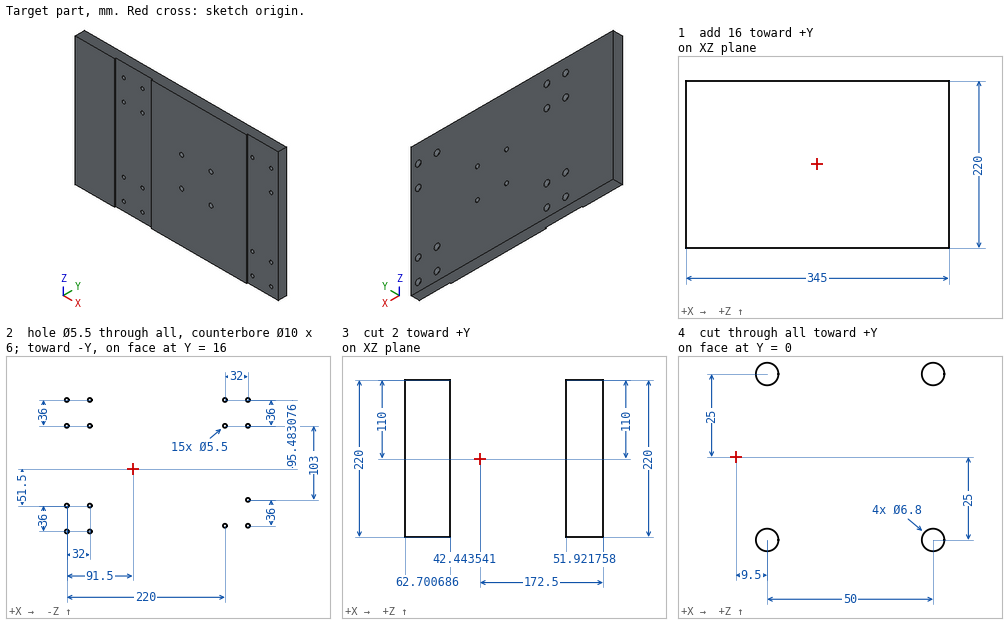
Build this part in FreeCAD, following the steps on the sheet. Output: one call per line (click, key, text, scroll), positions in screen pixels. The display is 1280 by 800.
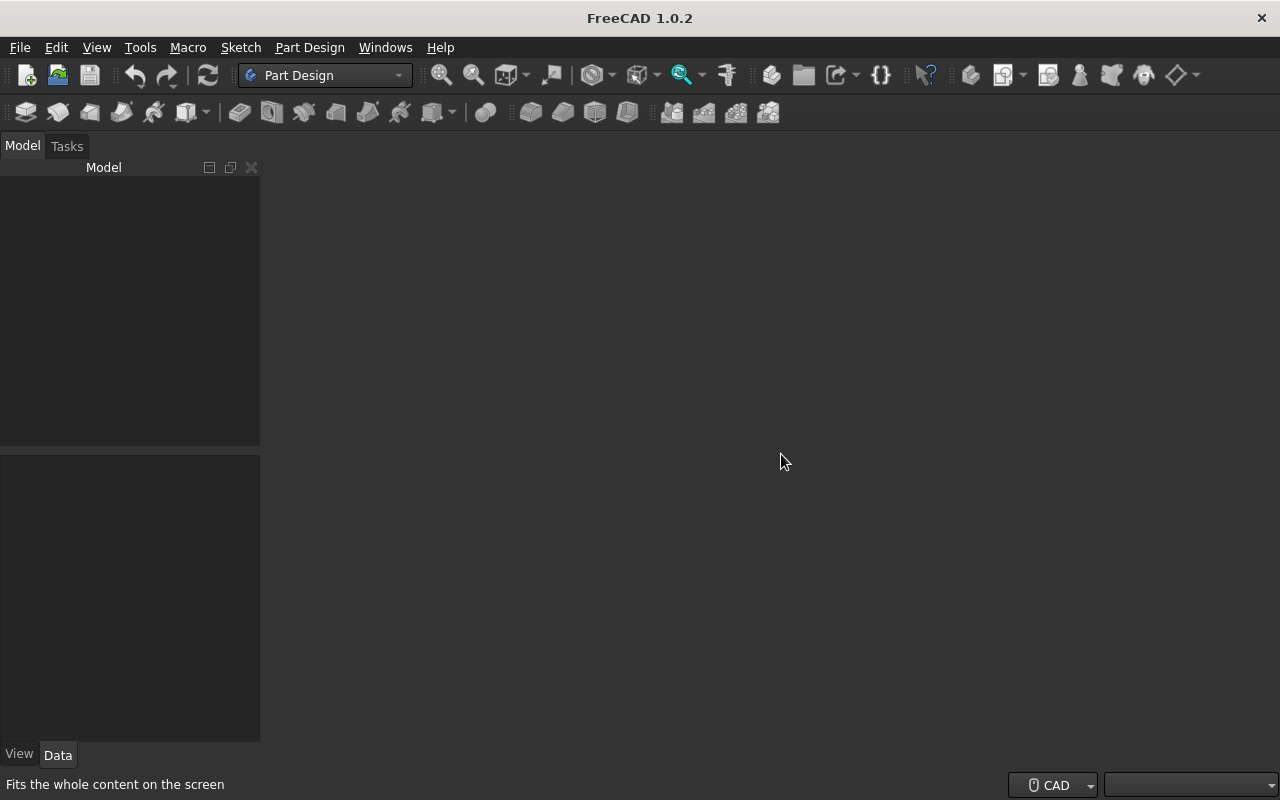
key(ctrl+n)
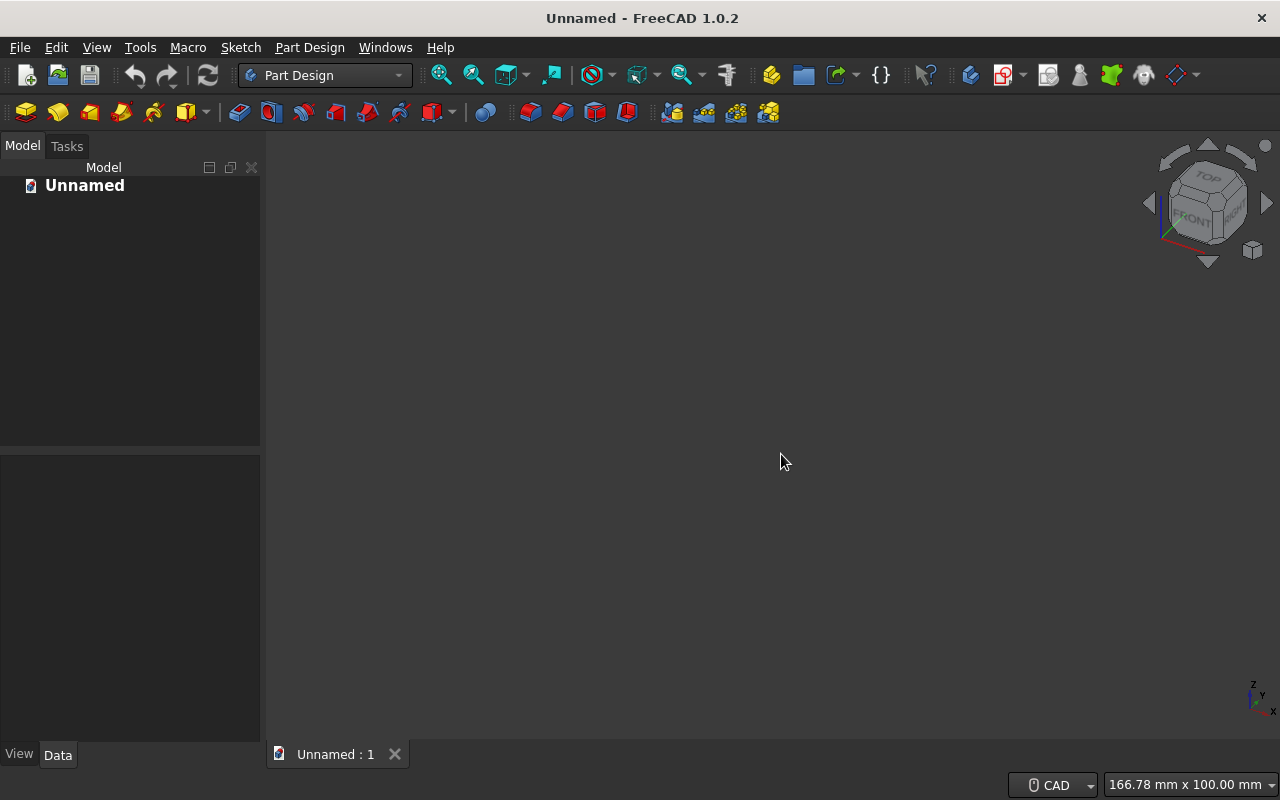
click(1004, 76)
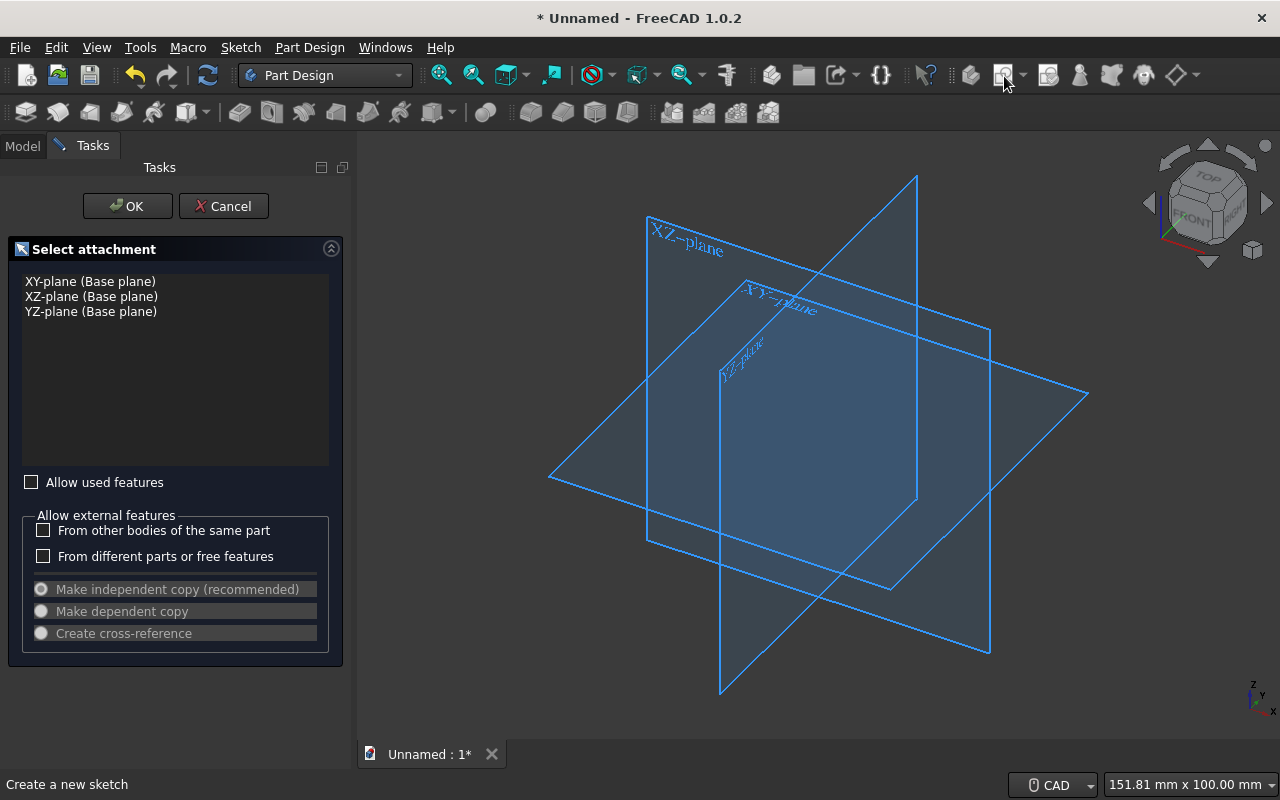
click(82, 296)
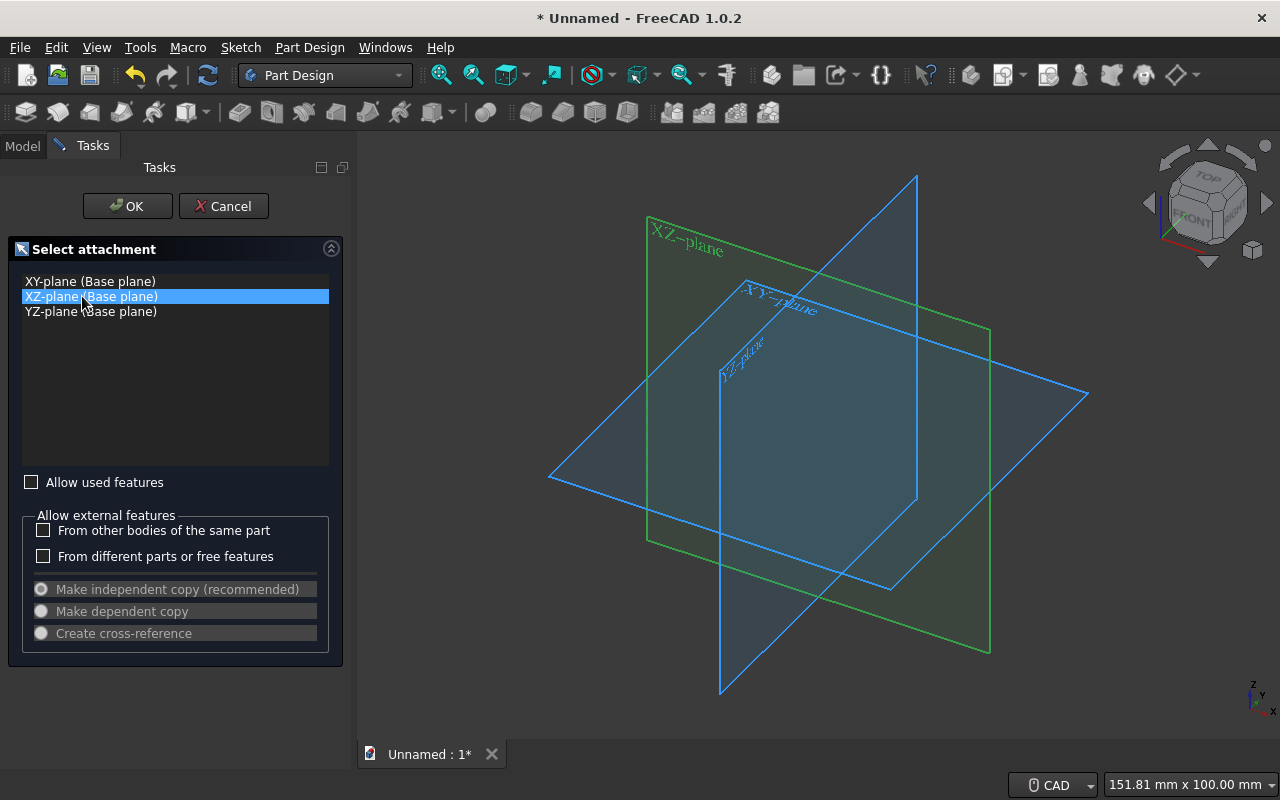
click(128, 206)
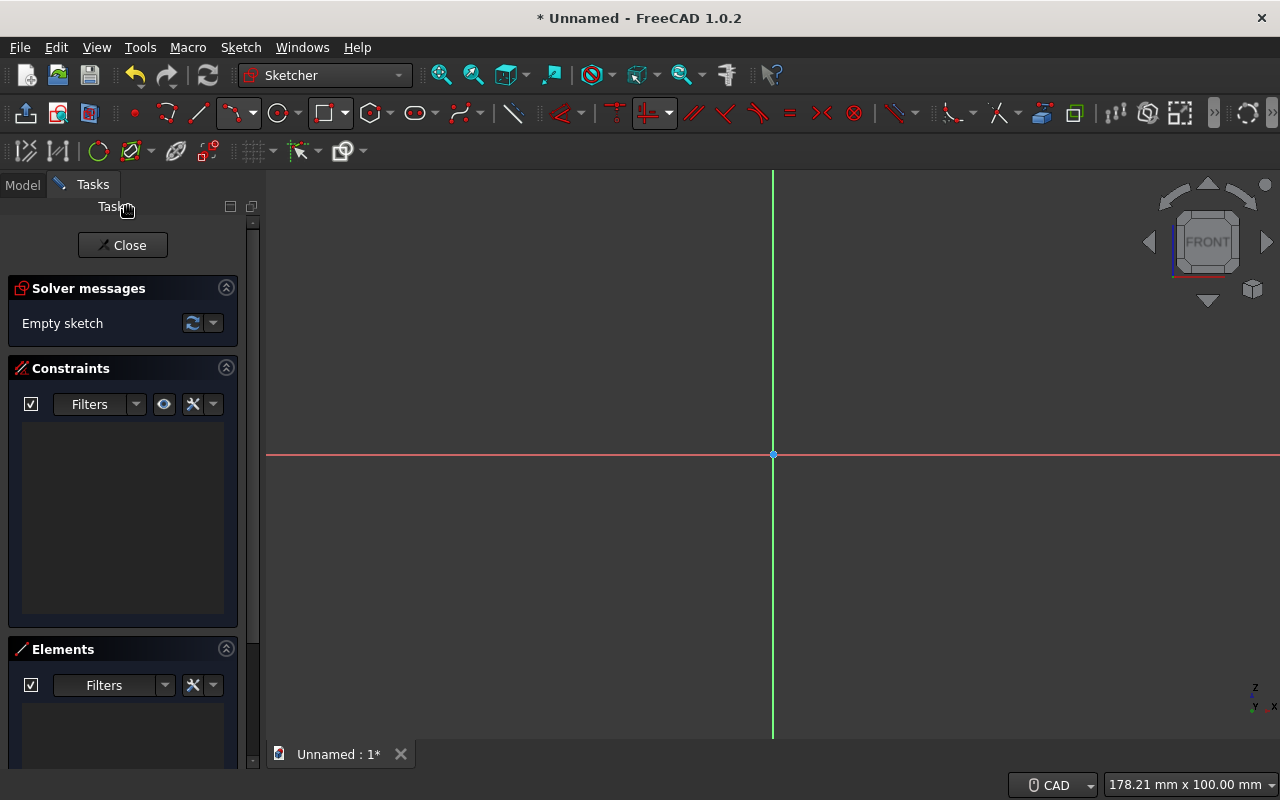
scroll(675, 454, down, 6)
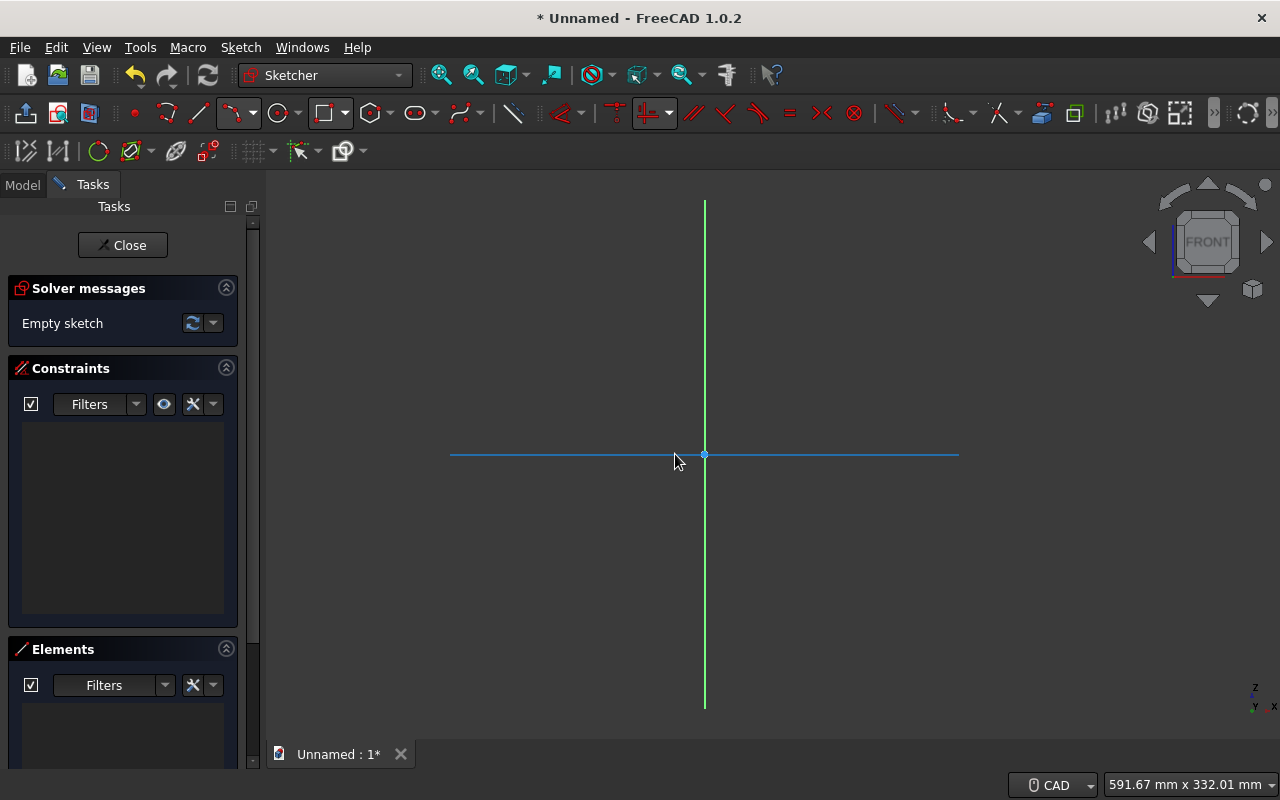
key(g)
key(v)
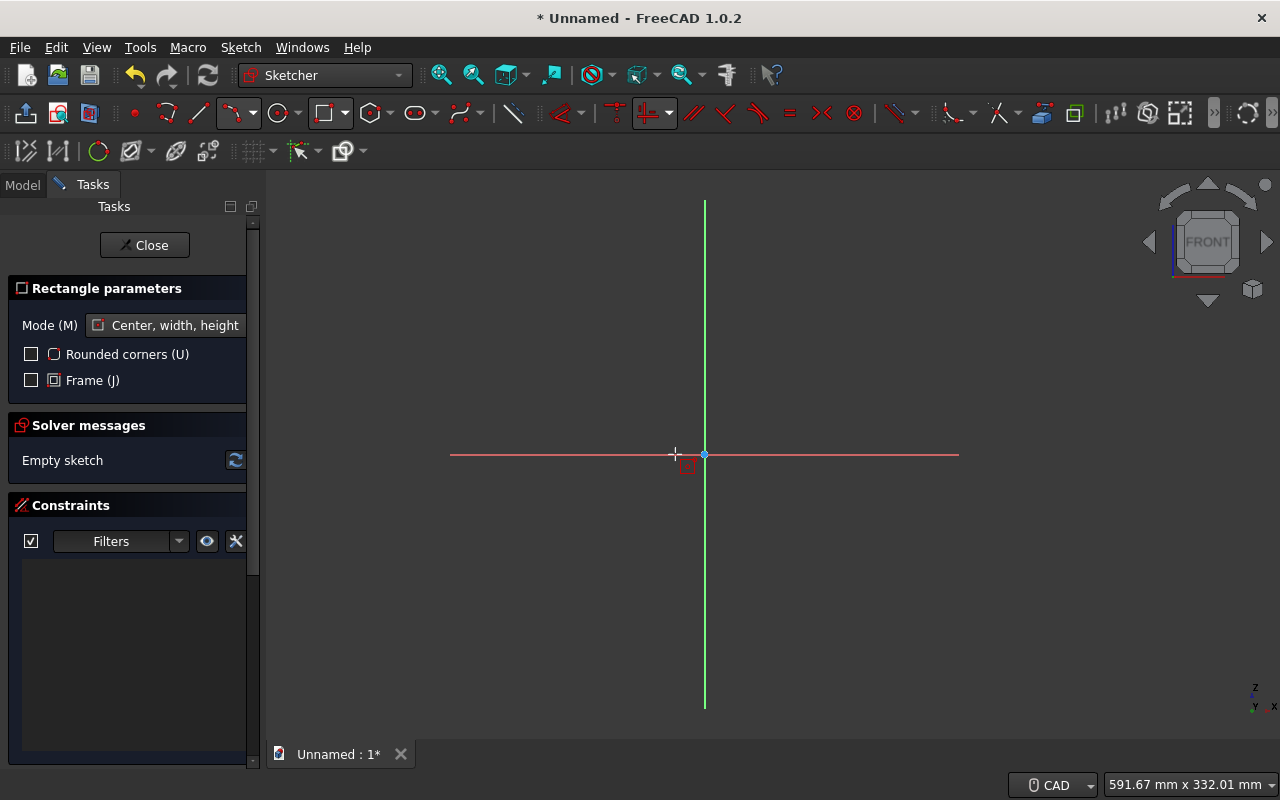
click(705, 454)
move(1000, 266)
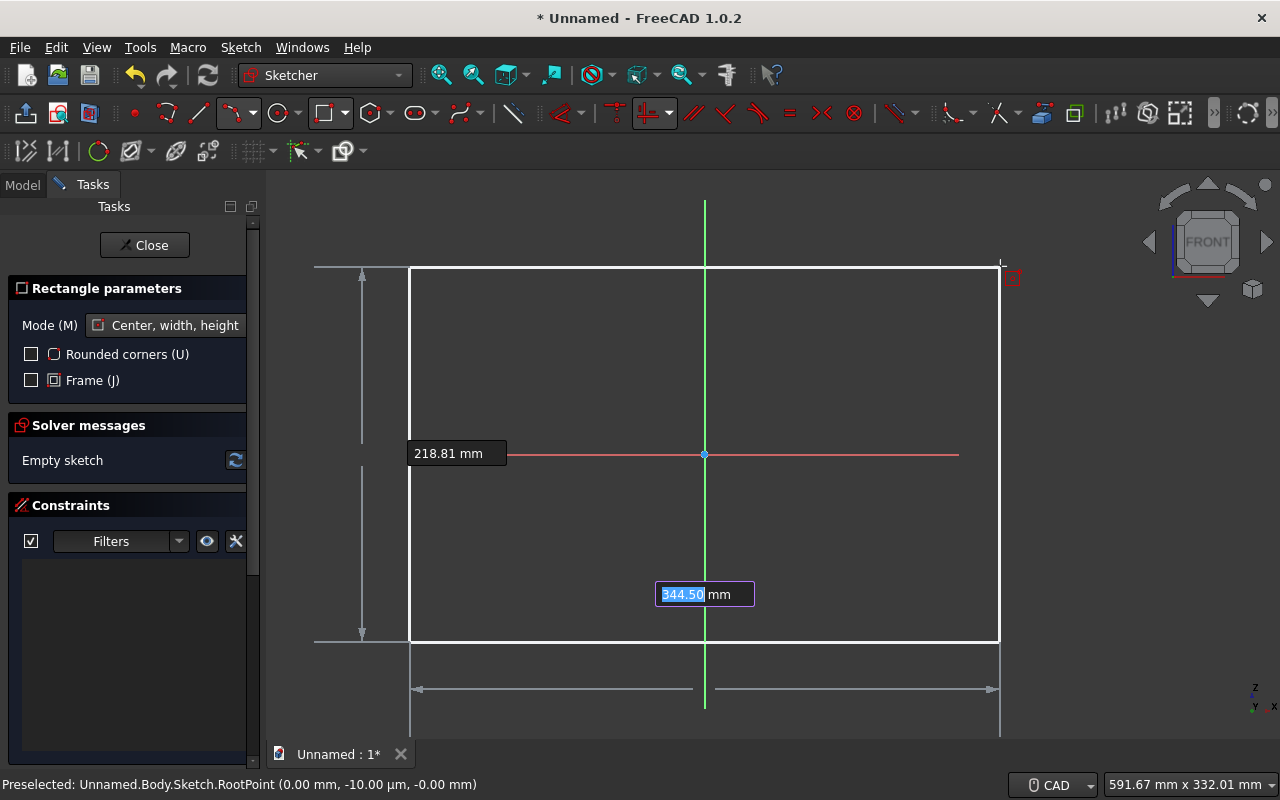
text(345)
key(Tab)
text(220)
key(Return)
key(Escape)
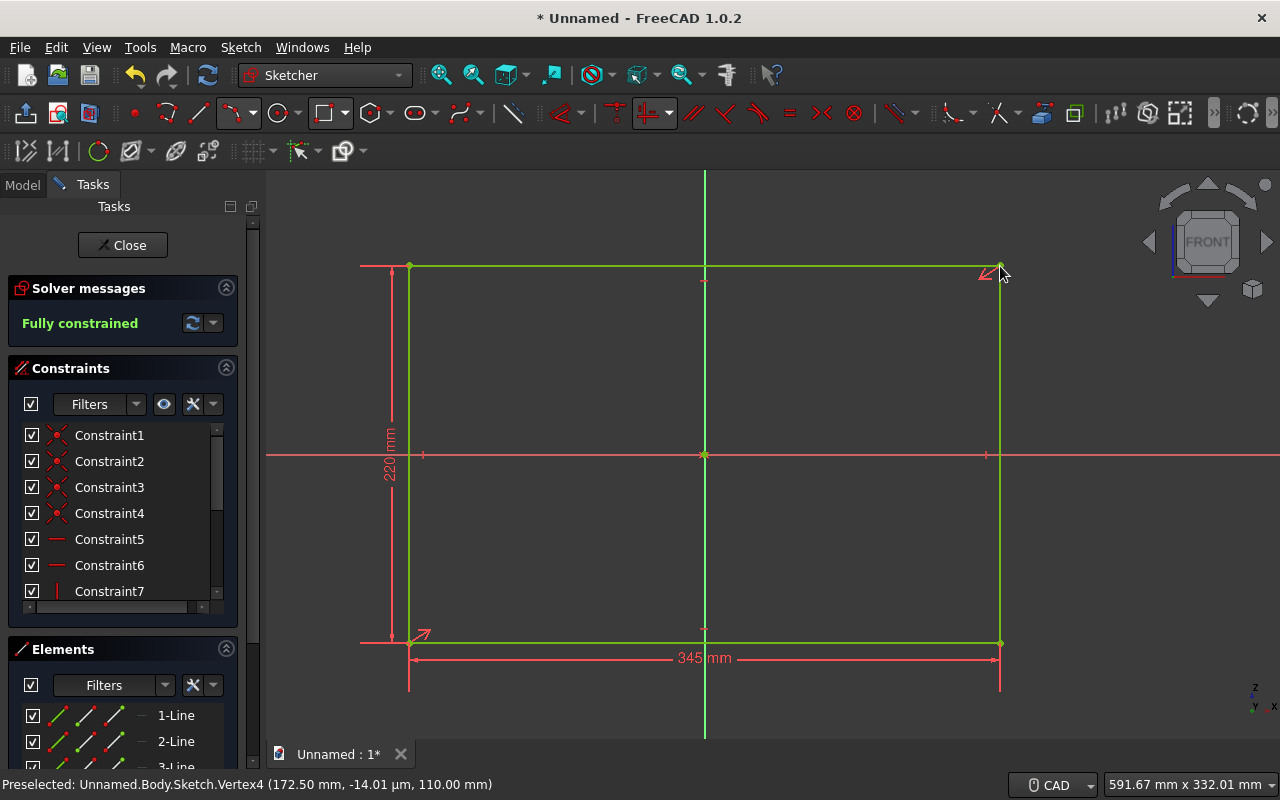
click(123, 245)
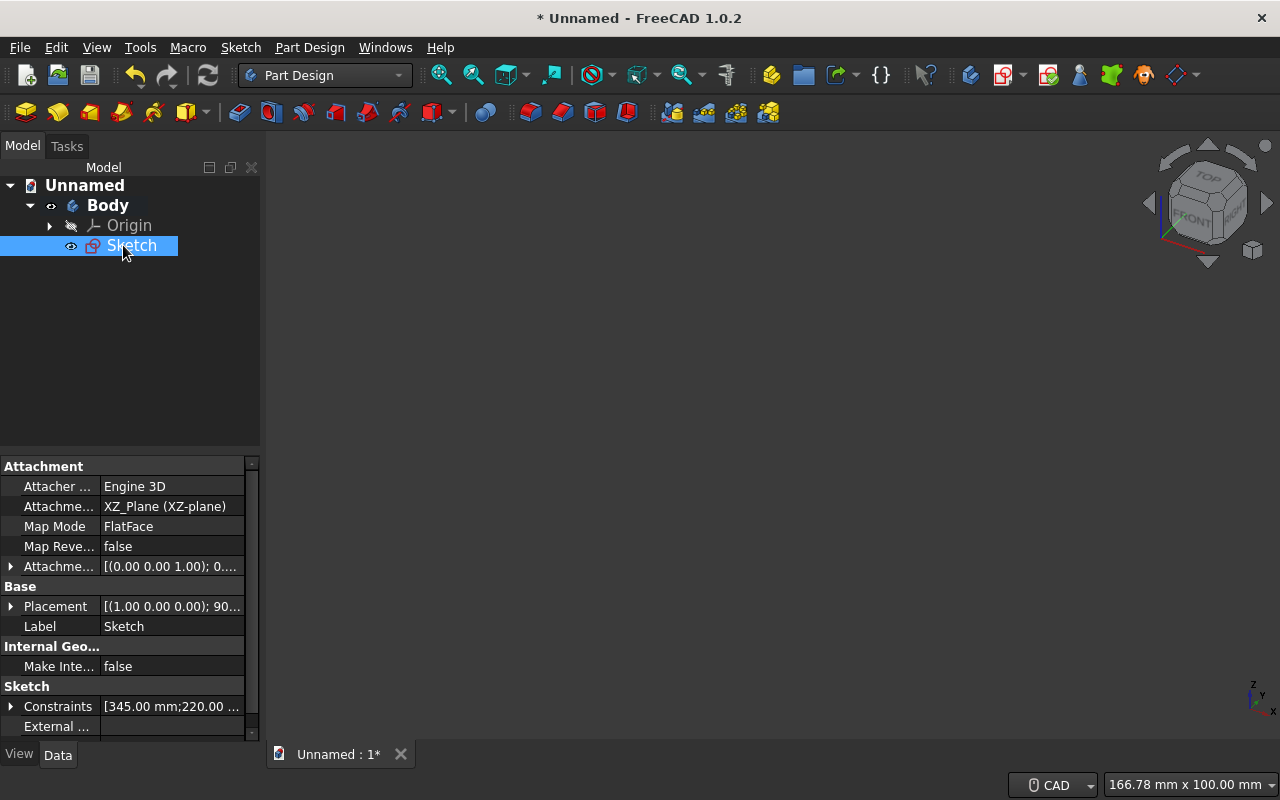
click(26, 112)